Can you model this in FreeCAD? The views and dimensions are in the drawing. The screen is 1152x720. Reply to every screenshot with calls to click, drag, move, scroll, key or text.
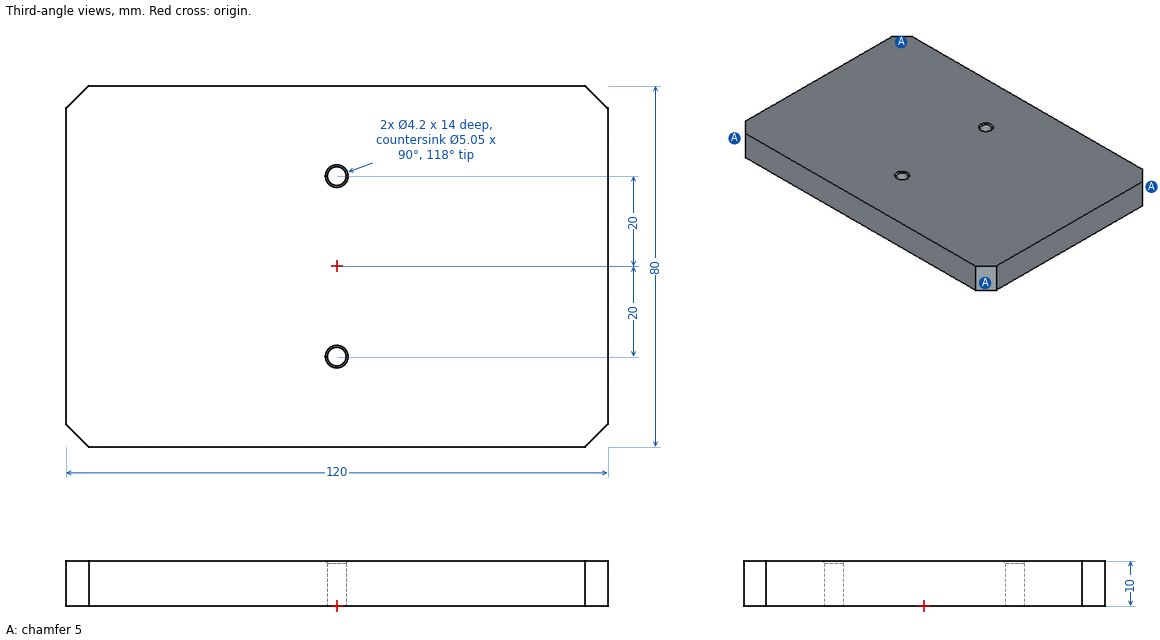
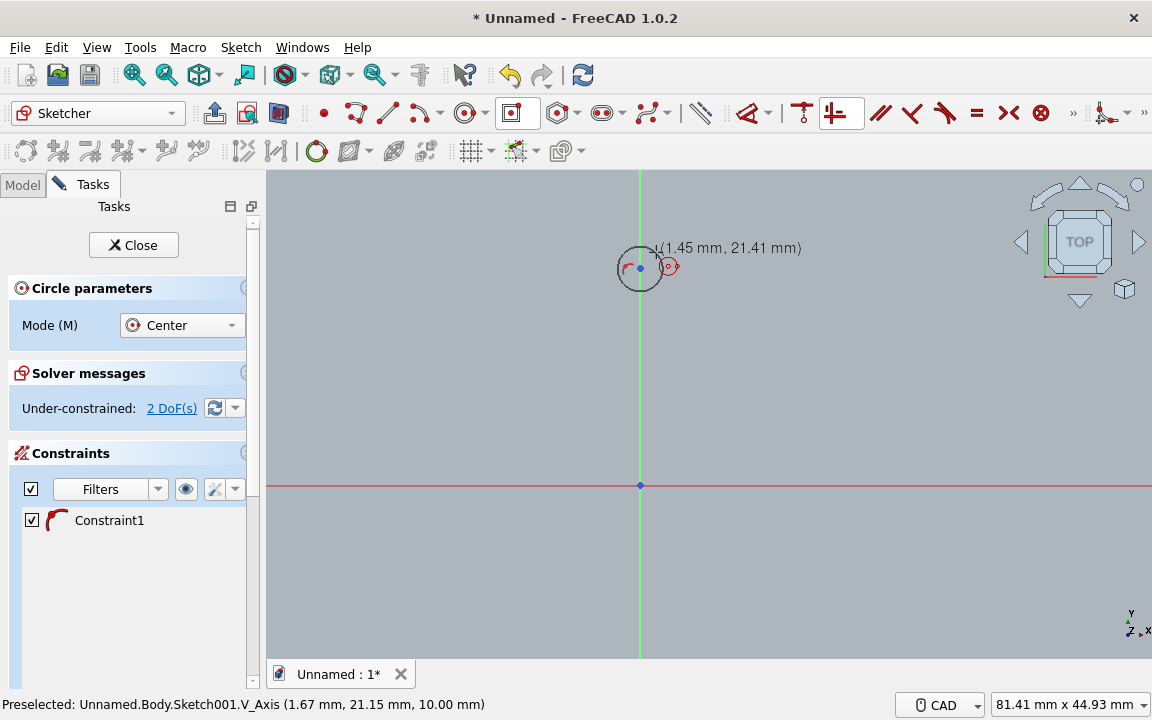
scroll(641, 269, down, 2)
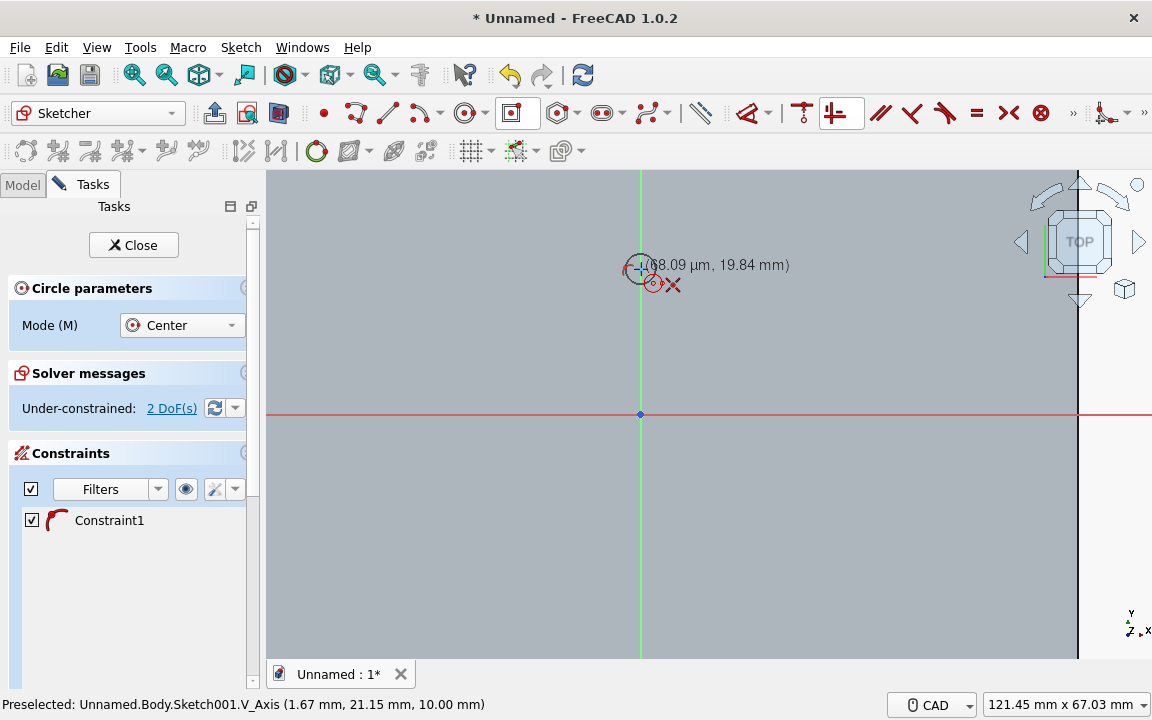
scroll(641, 560, up, 2)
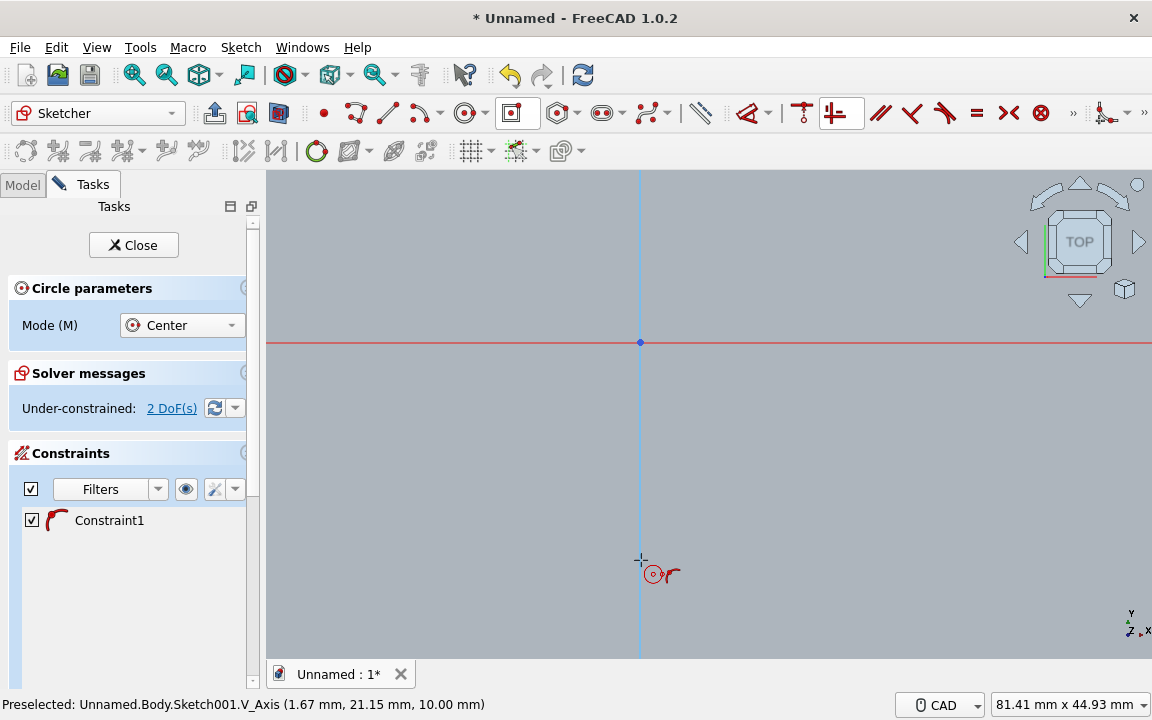
click(640, 560)
click(656, 544)
key(Escape)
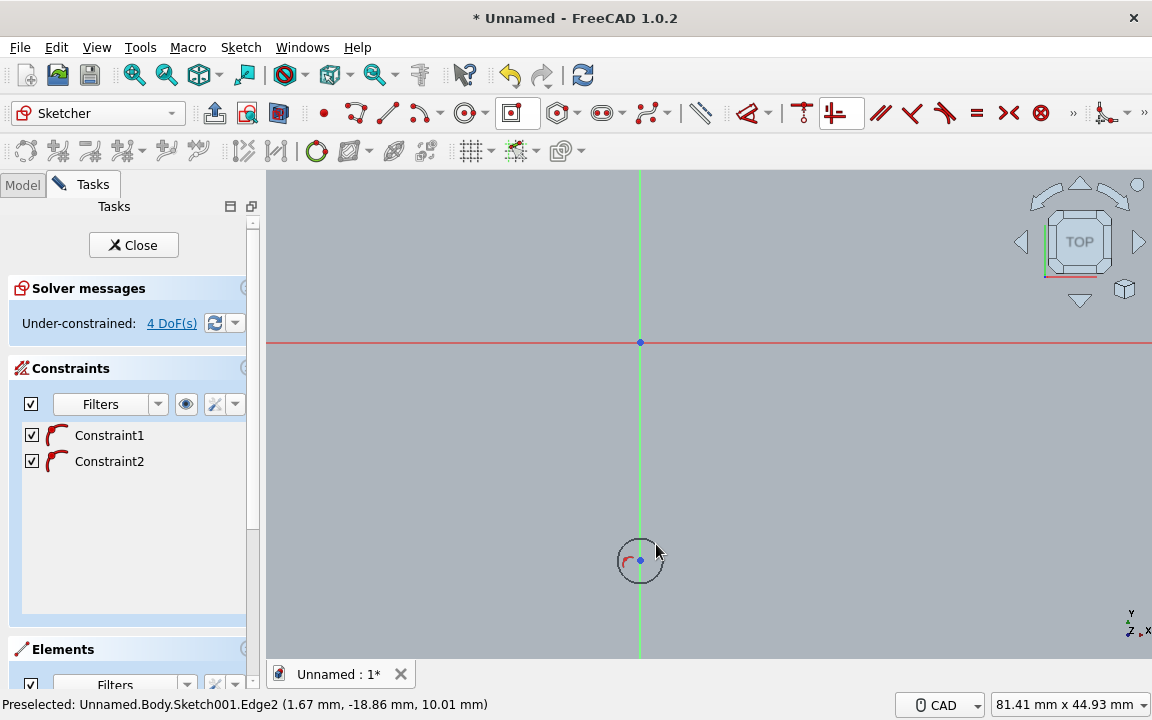
scroll(641, 561, down, 2)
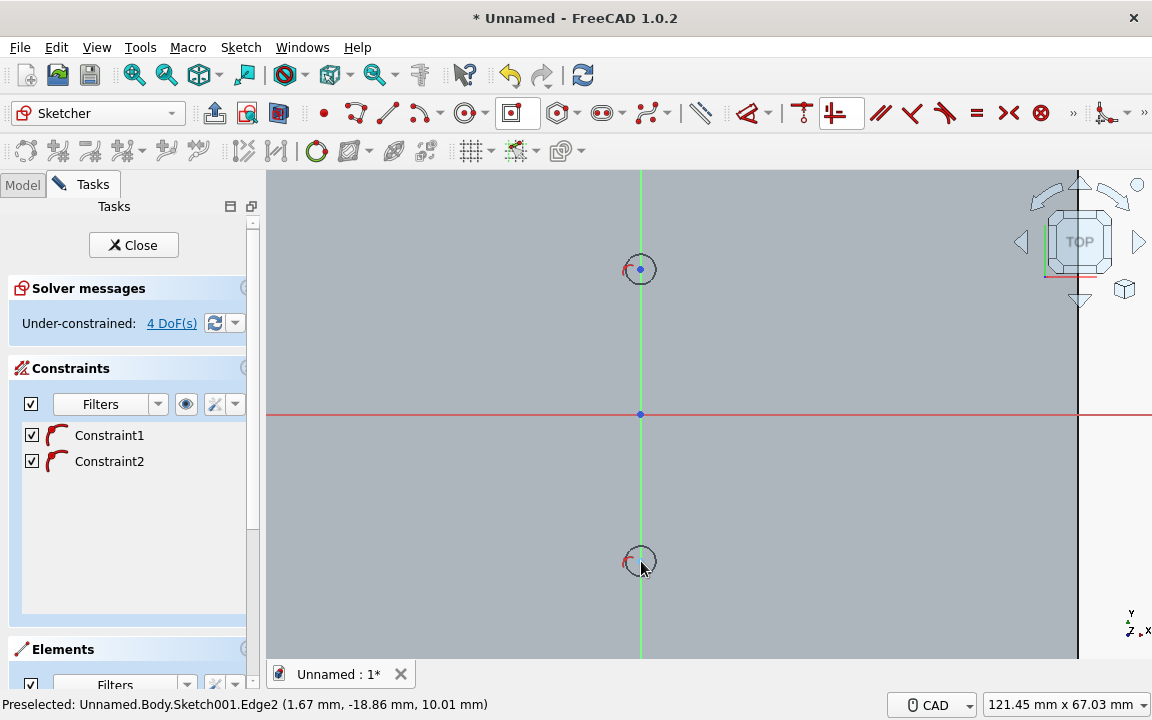
scroll(651, 259, up, 2)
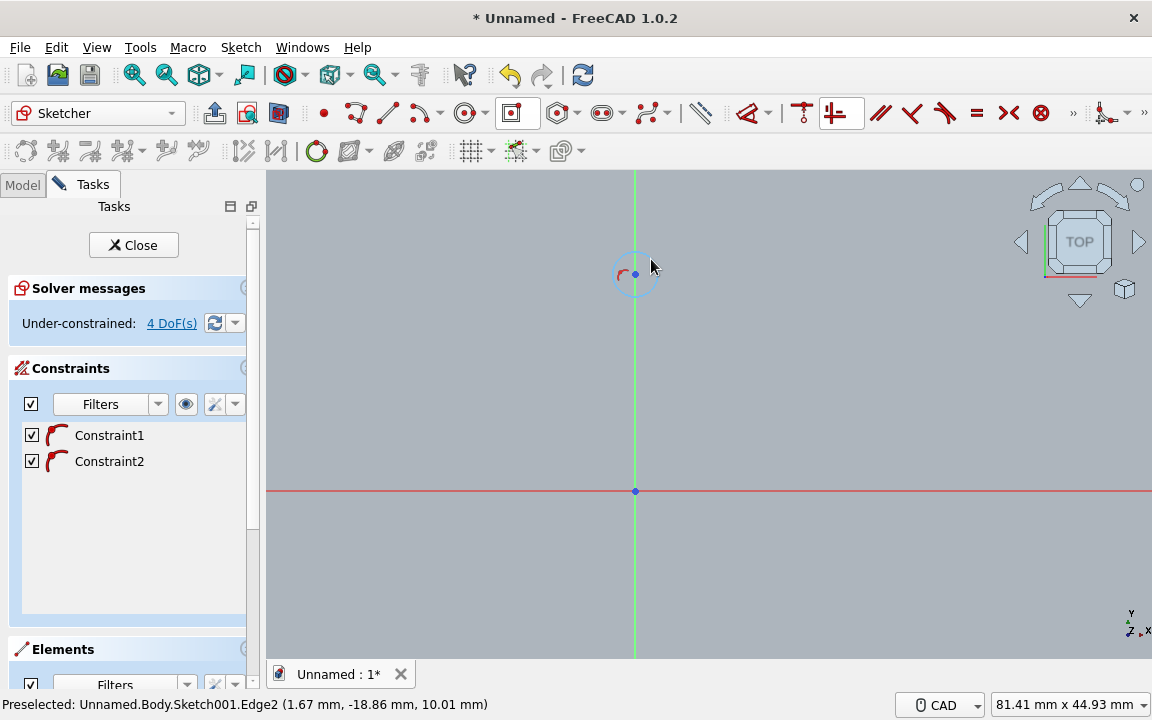
click(651, 259)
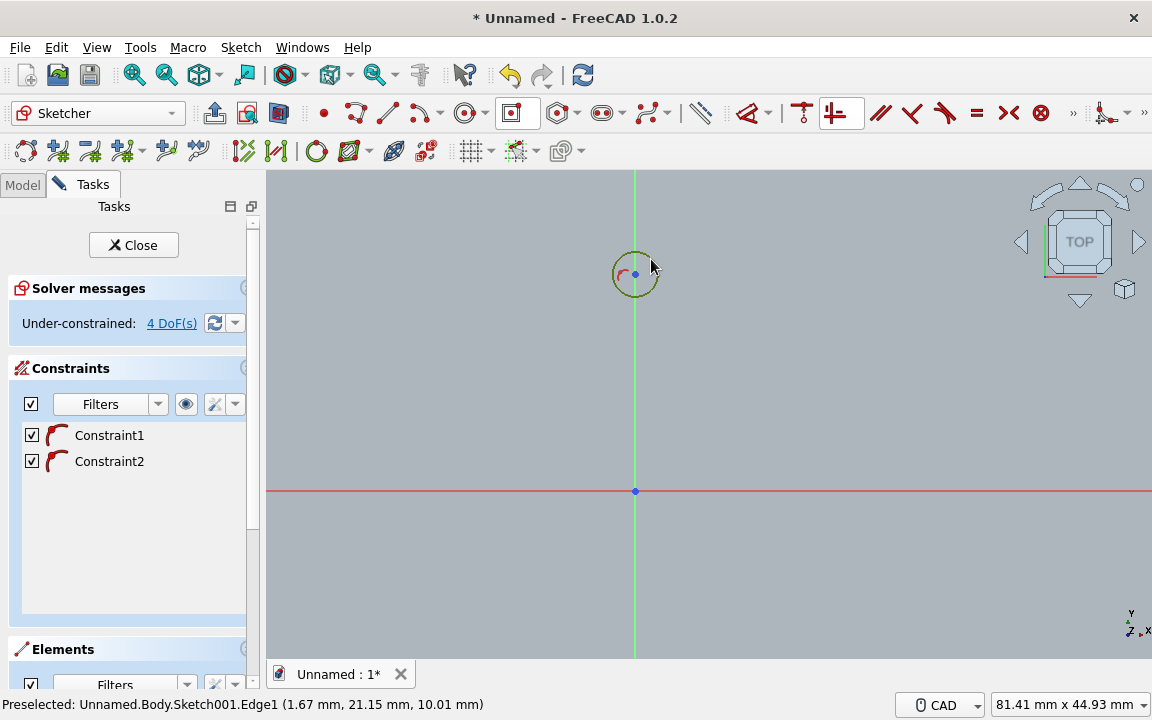
scroll(651, 258, down, 2)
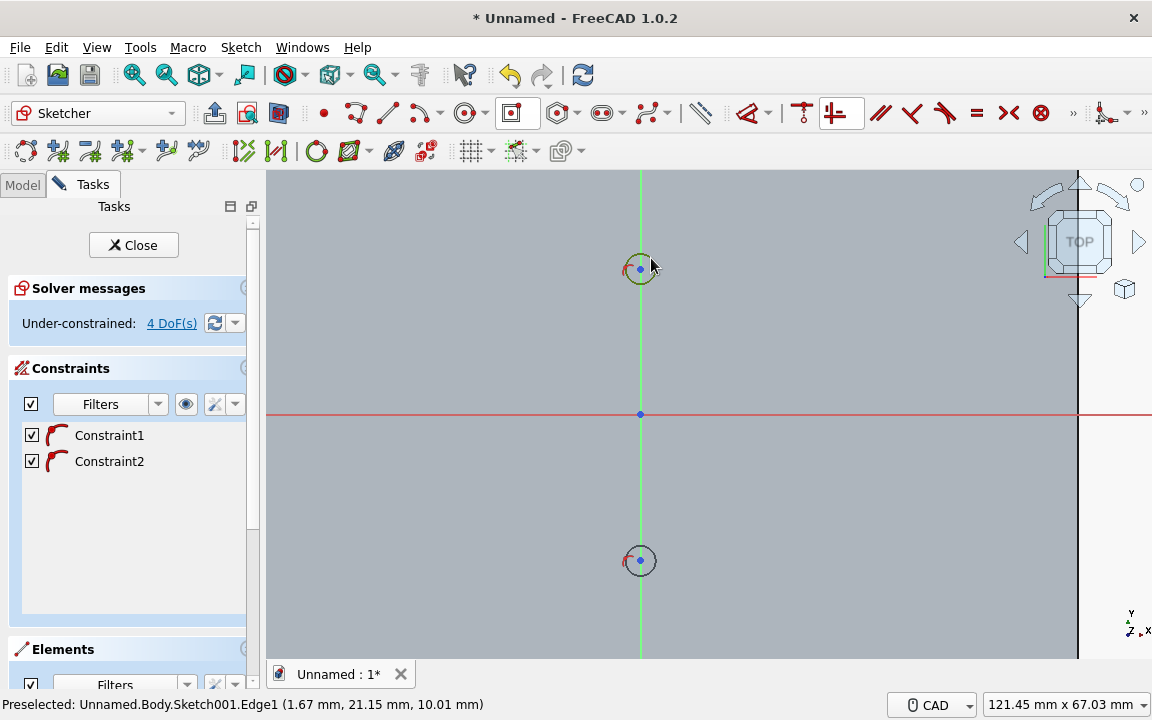
scroll(651, 550, up, 2)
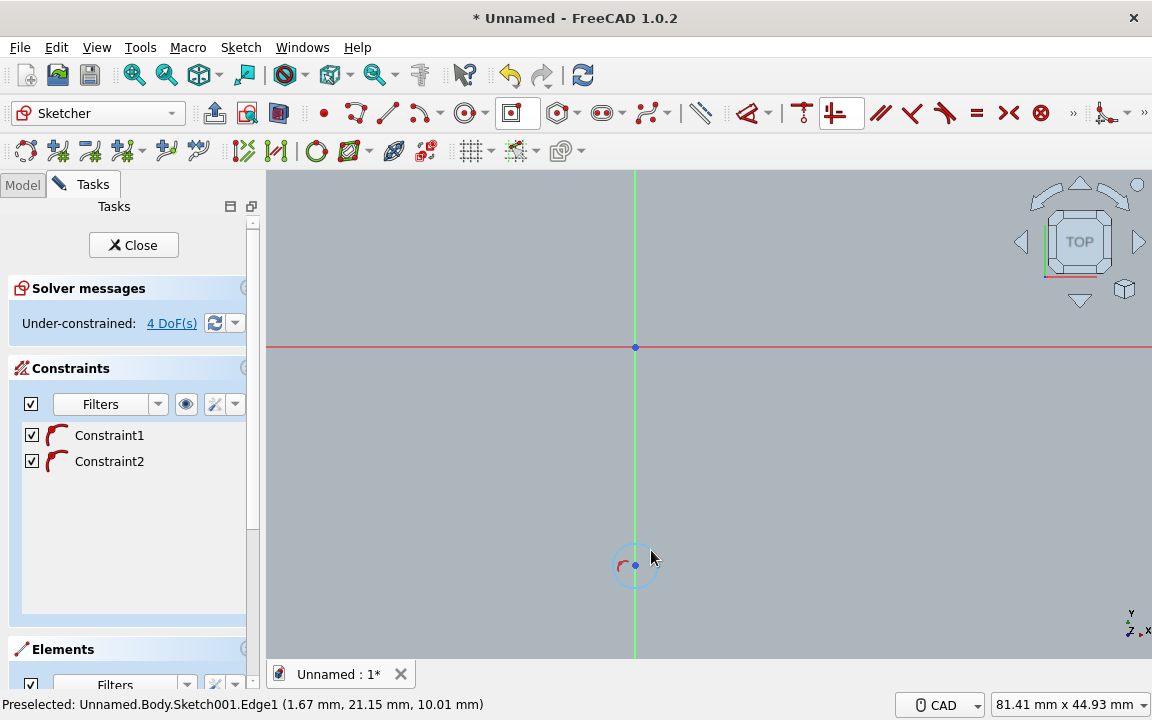
click(651, 550)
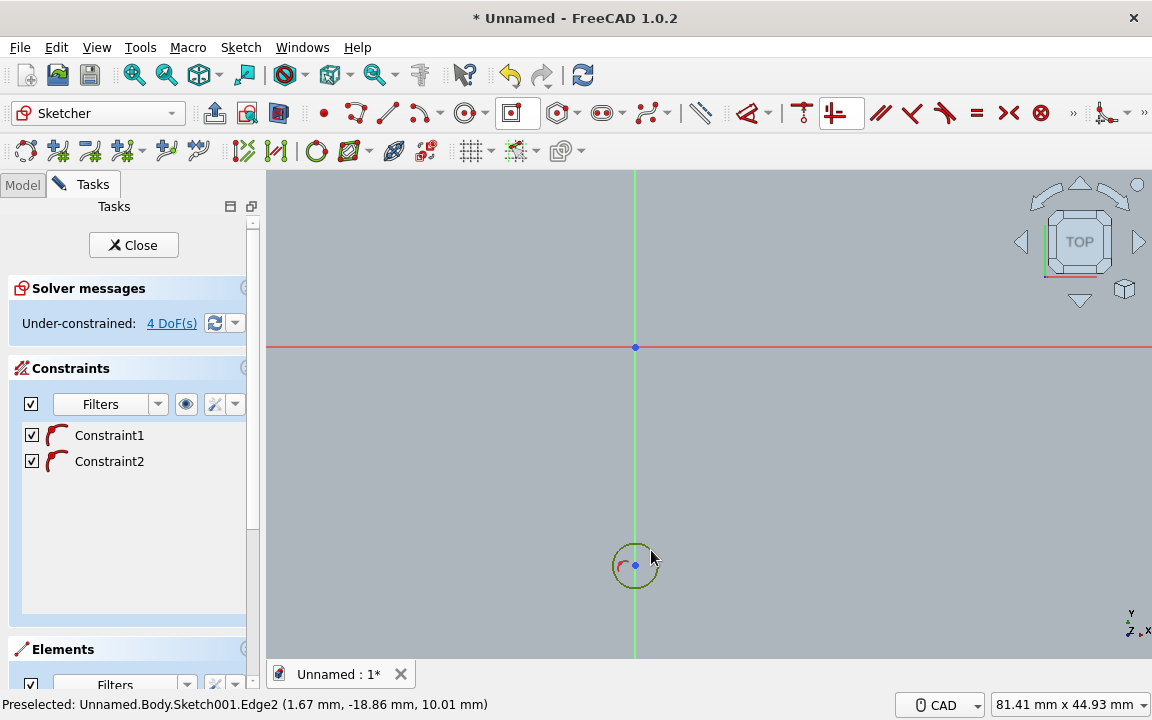
key(e)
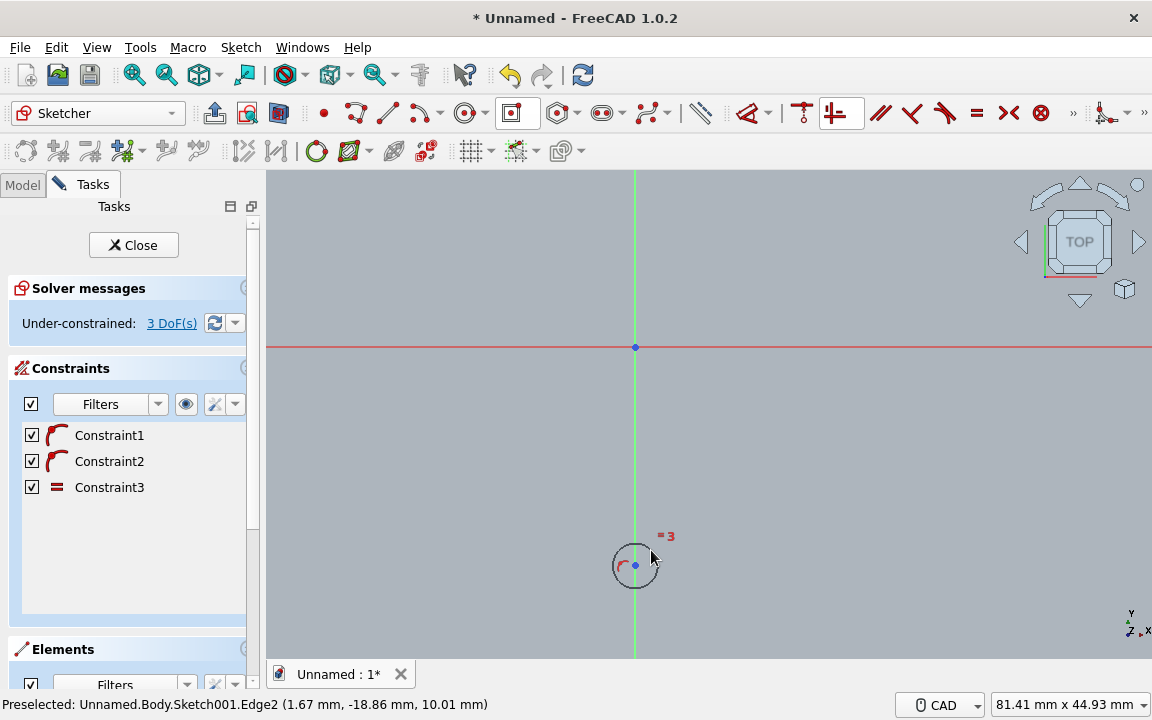
key(d)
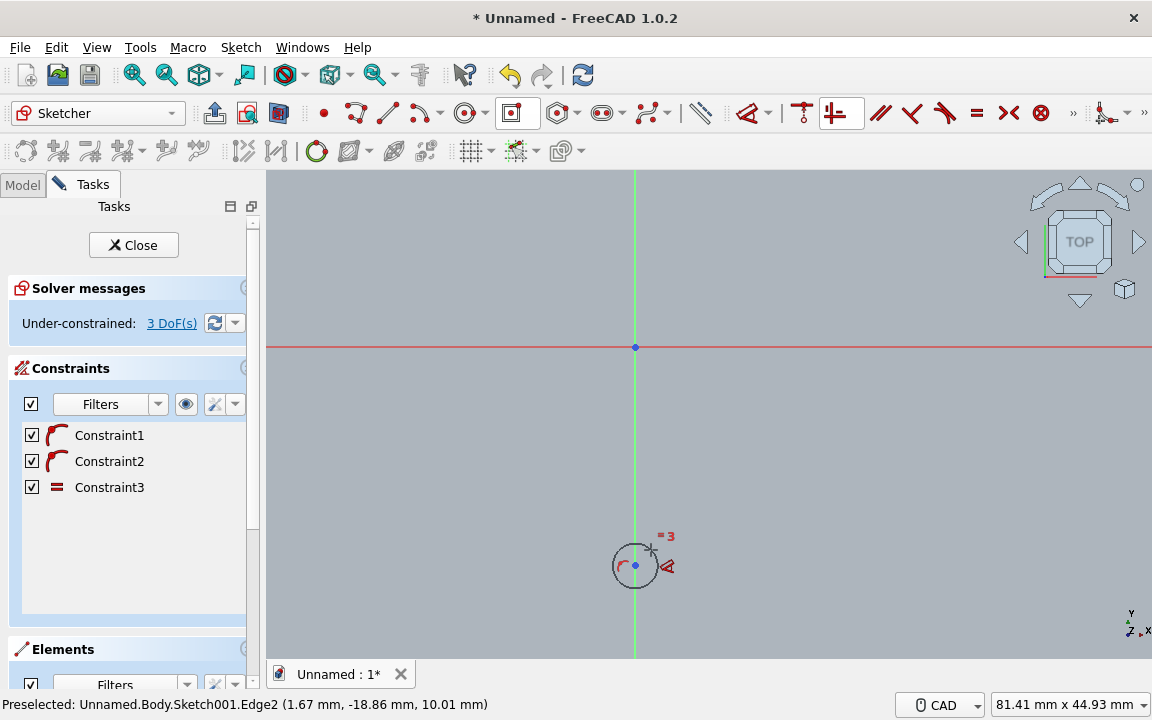
scroll(651, 551, down, 2)